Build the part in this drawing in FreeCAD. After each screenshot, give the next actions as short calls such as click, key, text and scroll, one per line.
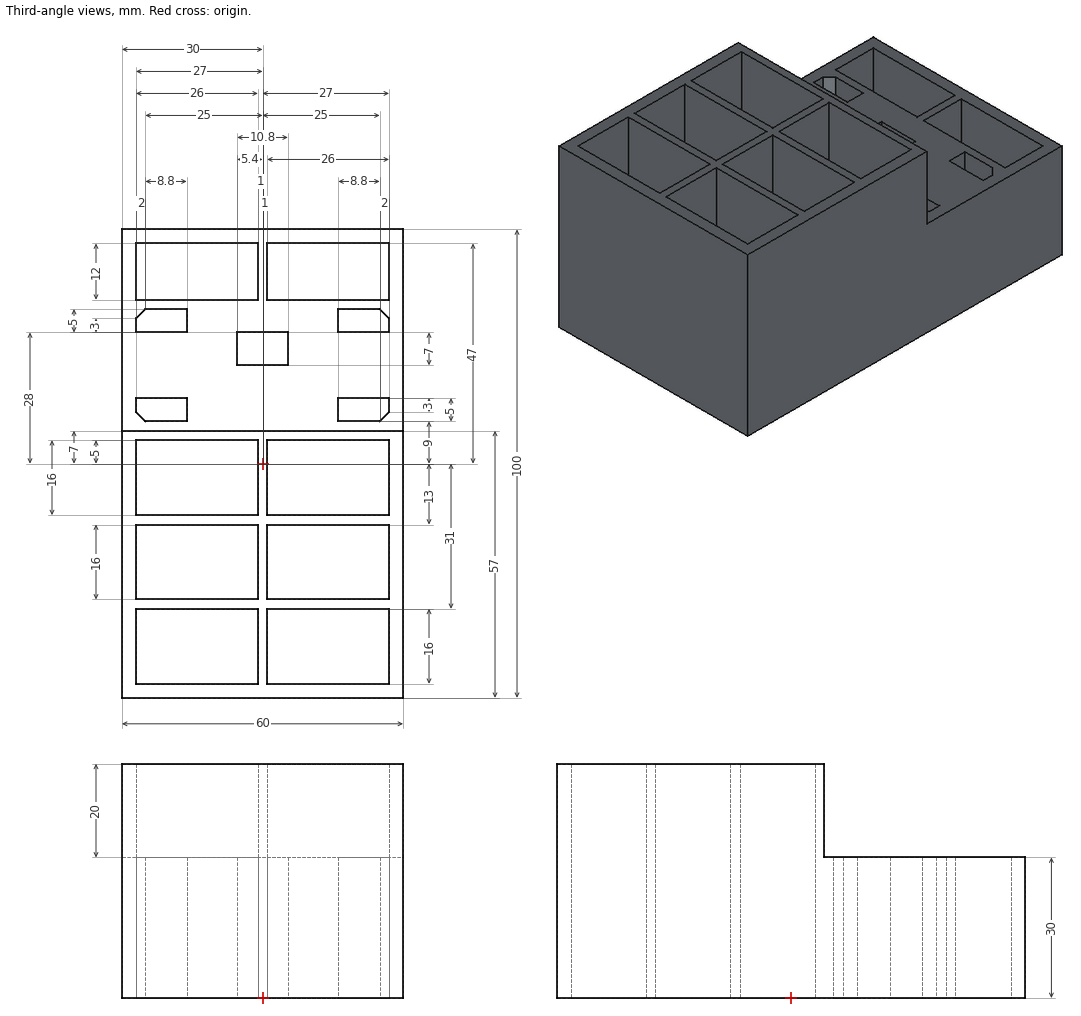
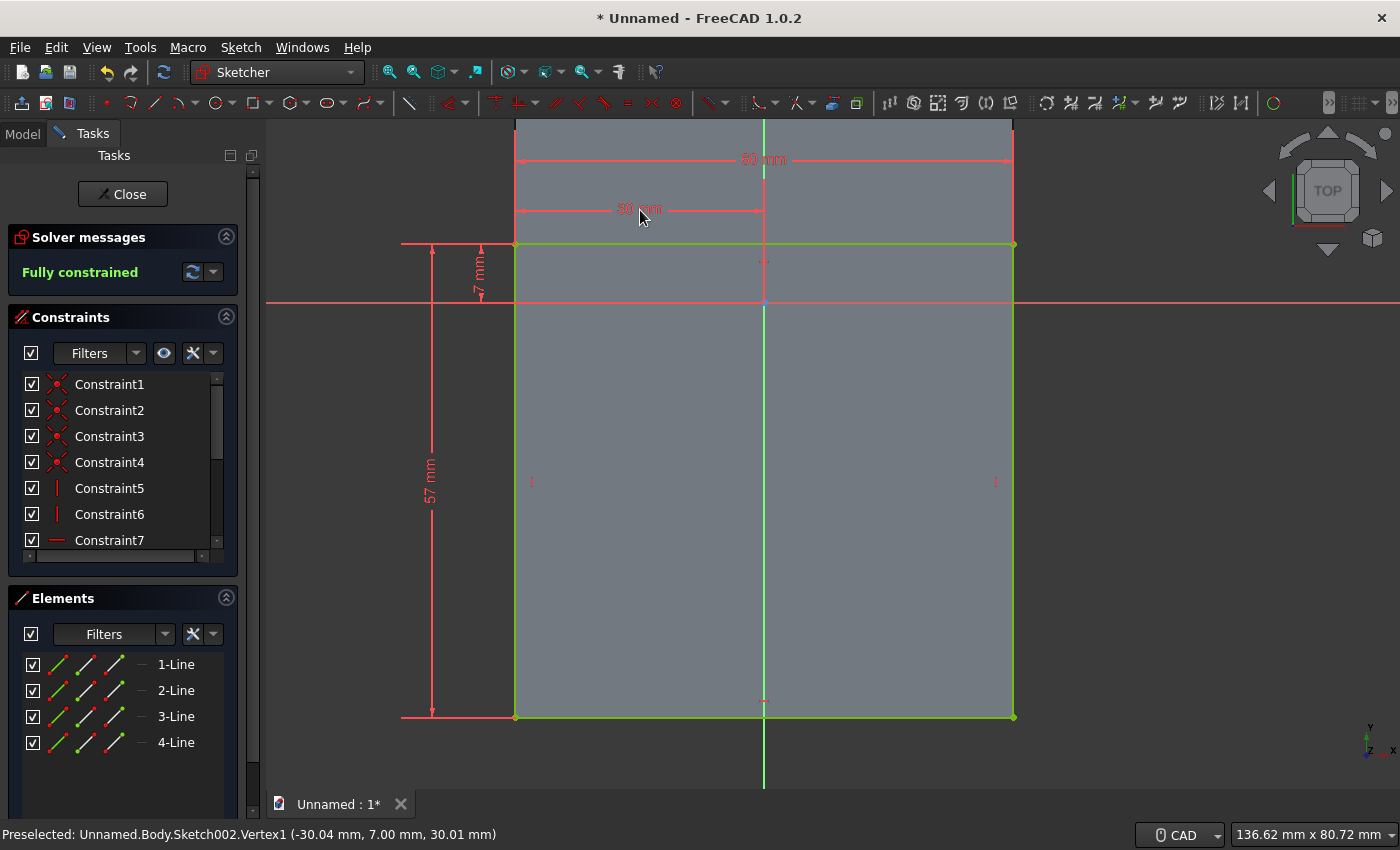
click(123, 194)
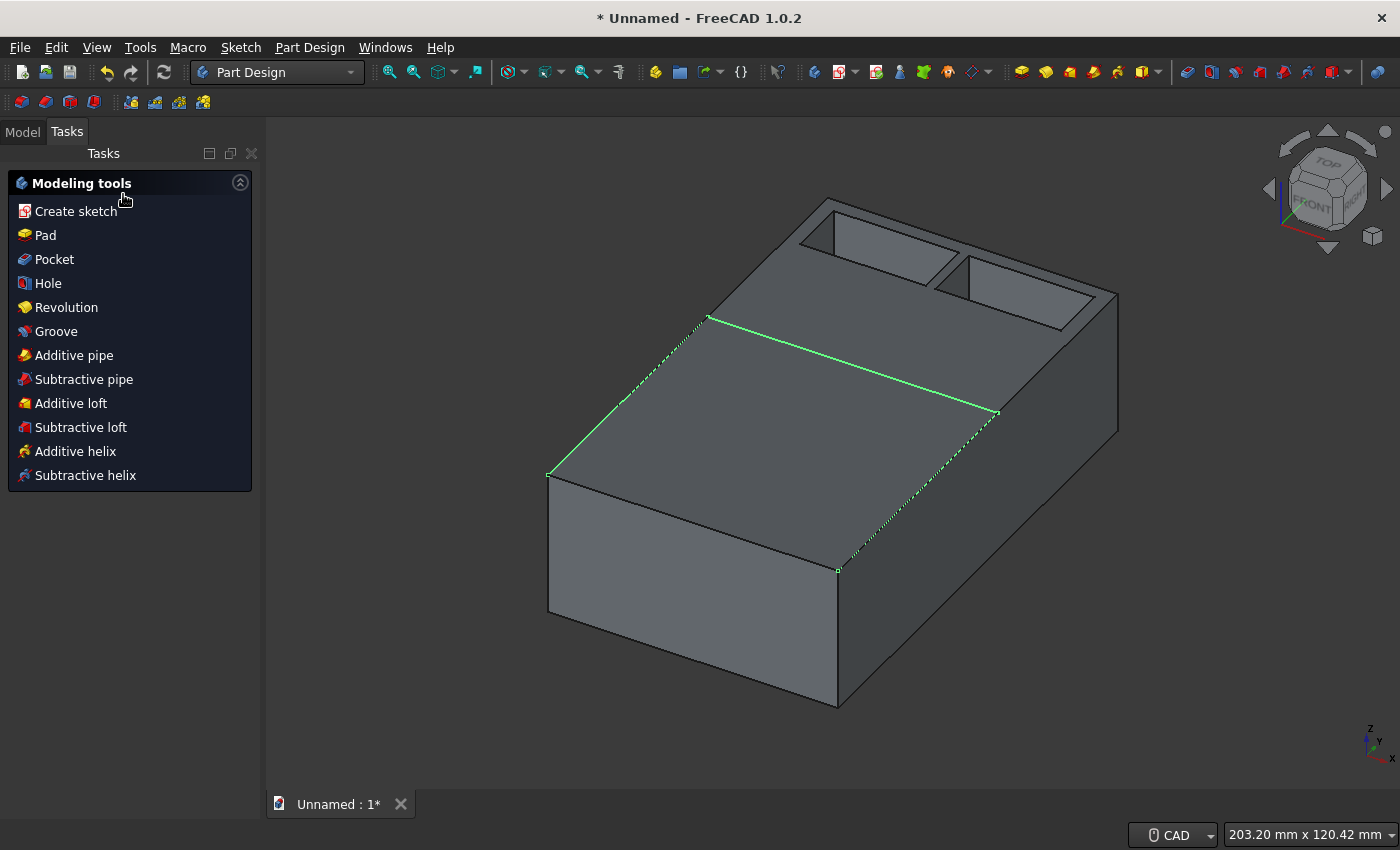
click(1022, 72)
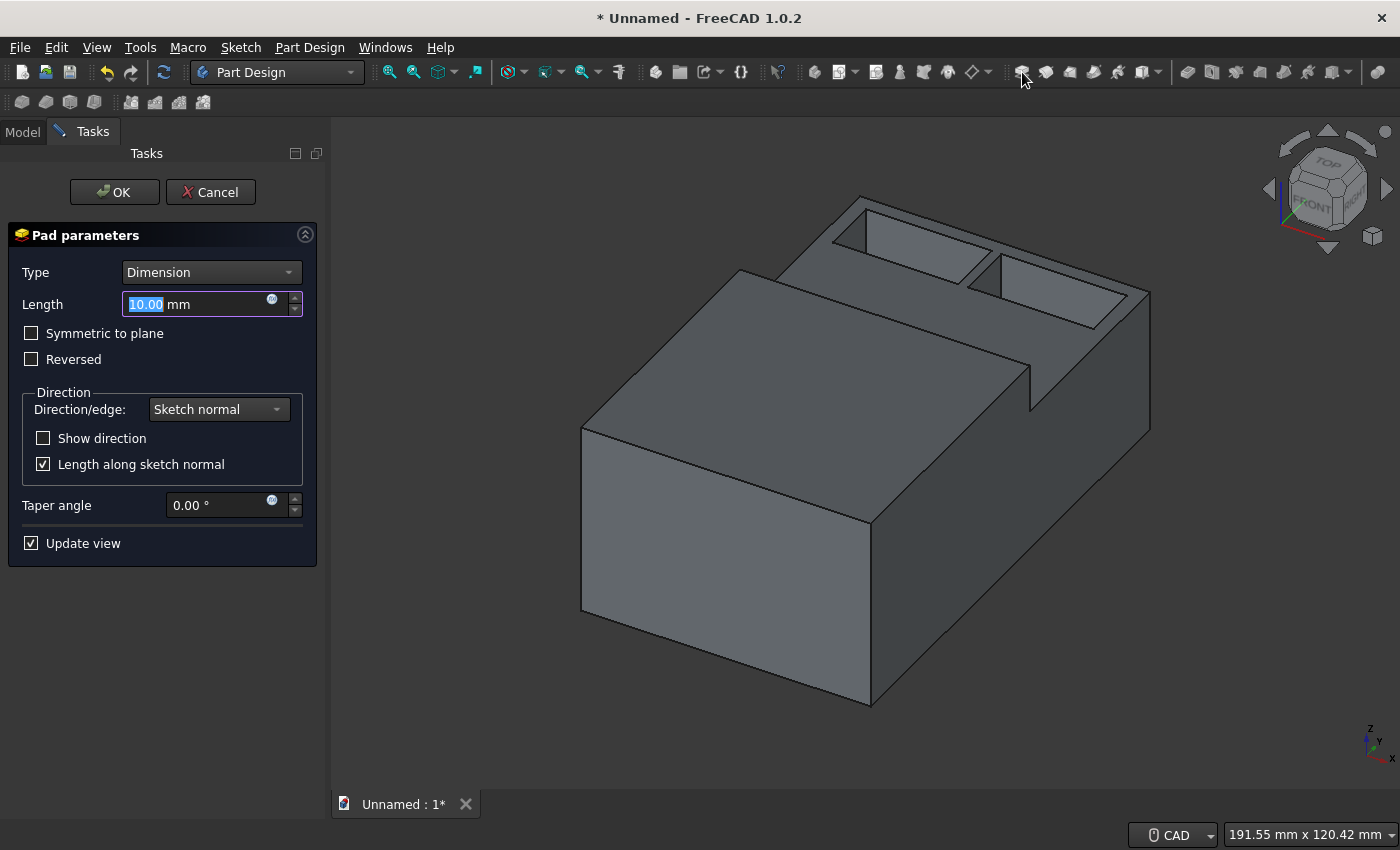
text(20)
key(Tab)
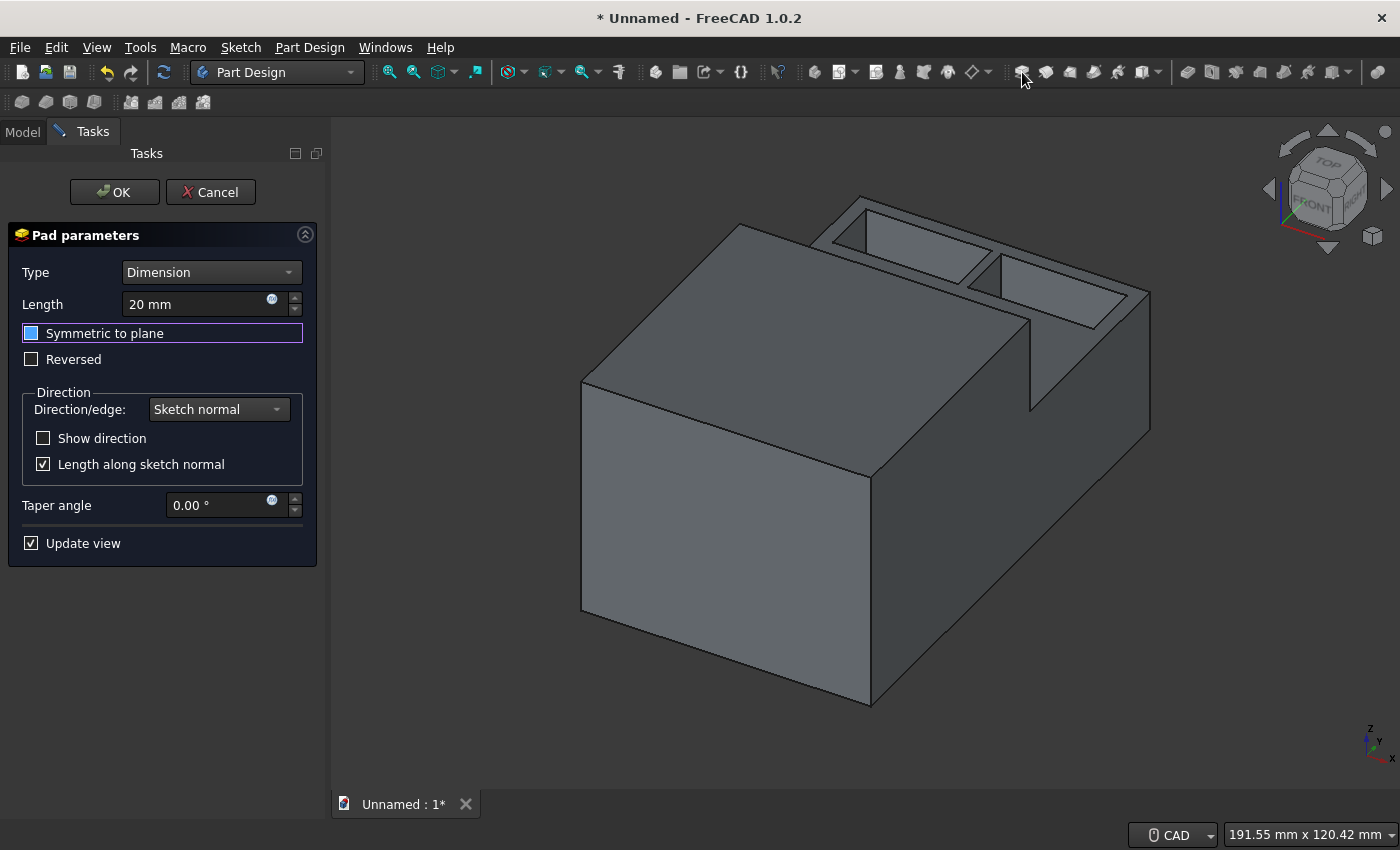
click(115, 192)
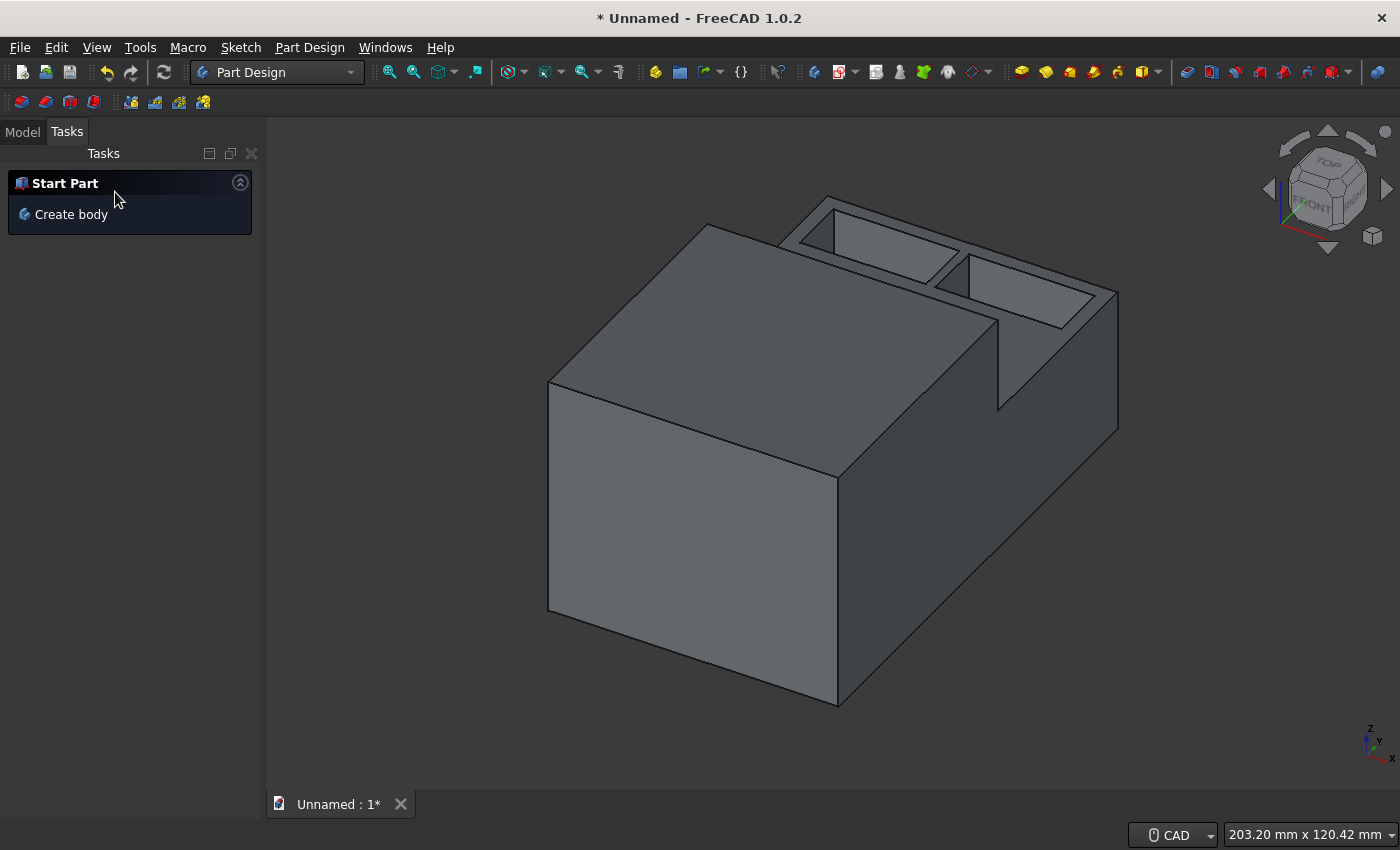
key(v)
key(f)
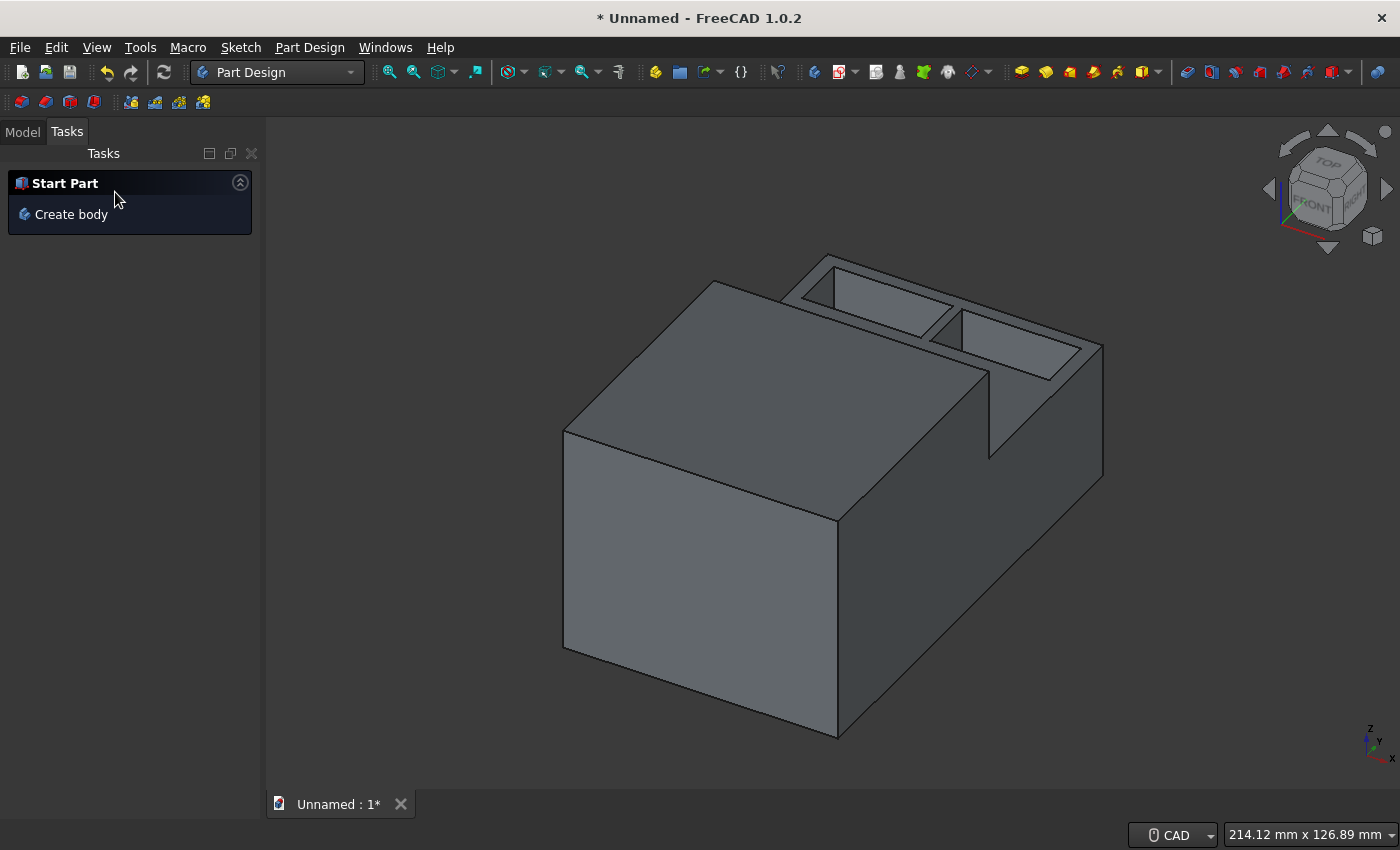
click(776, 400)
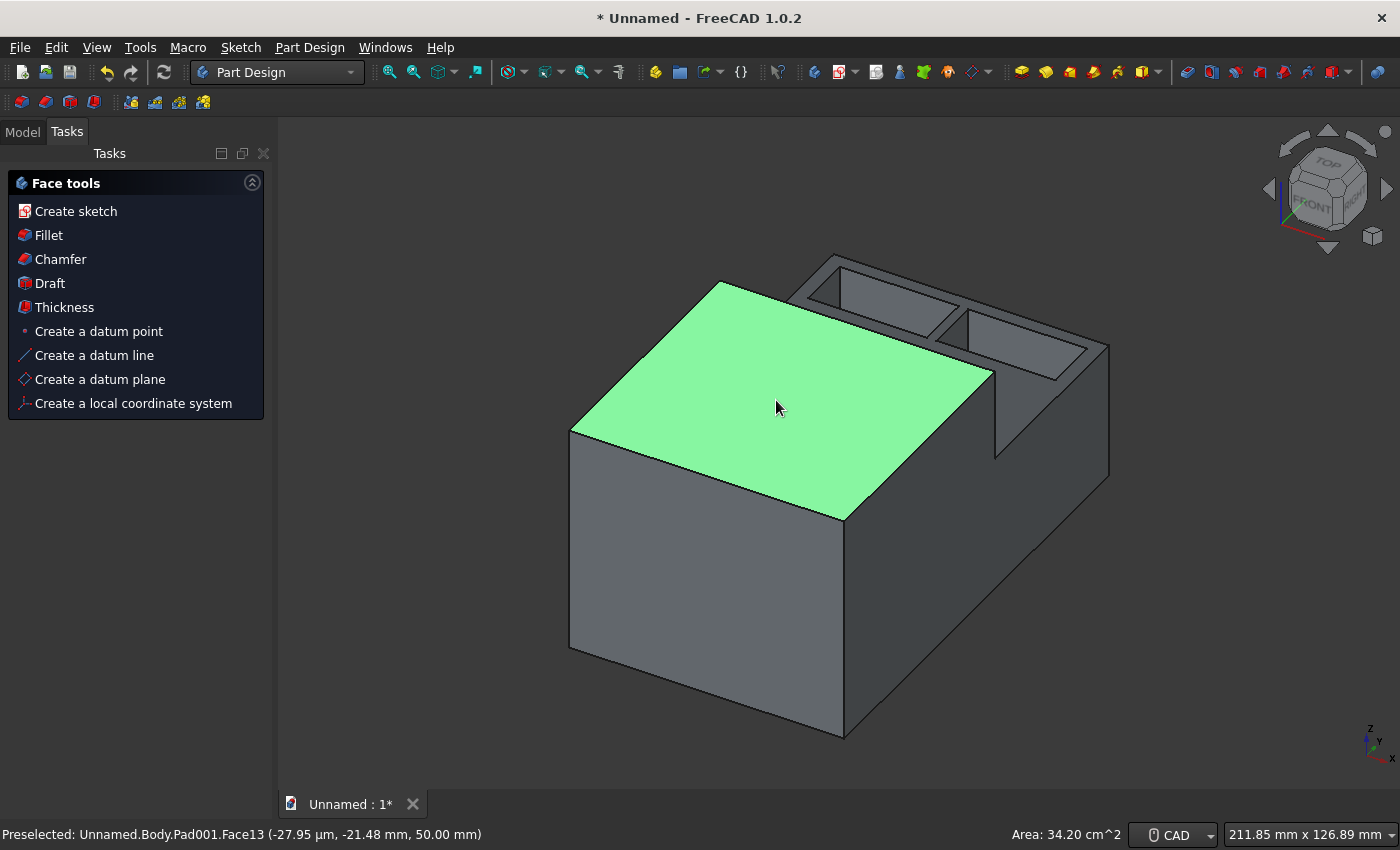
click(840, 72)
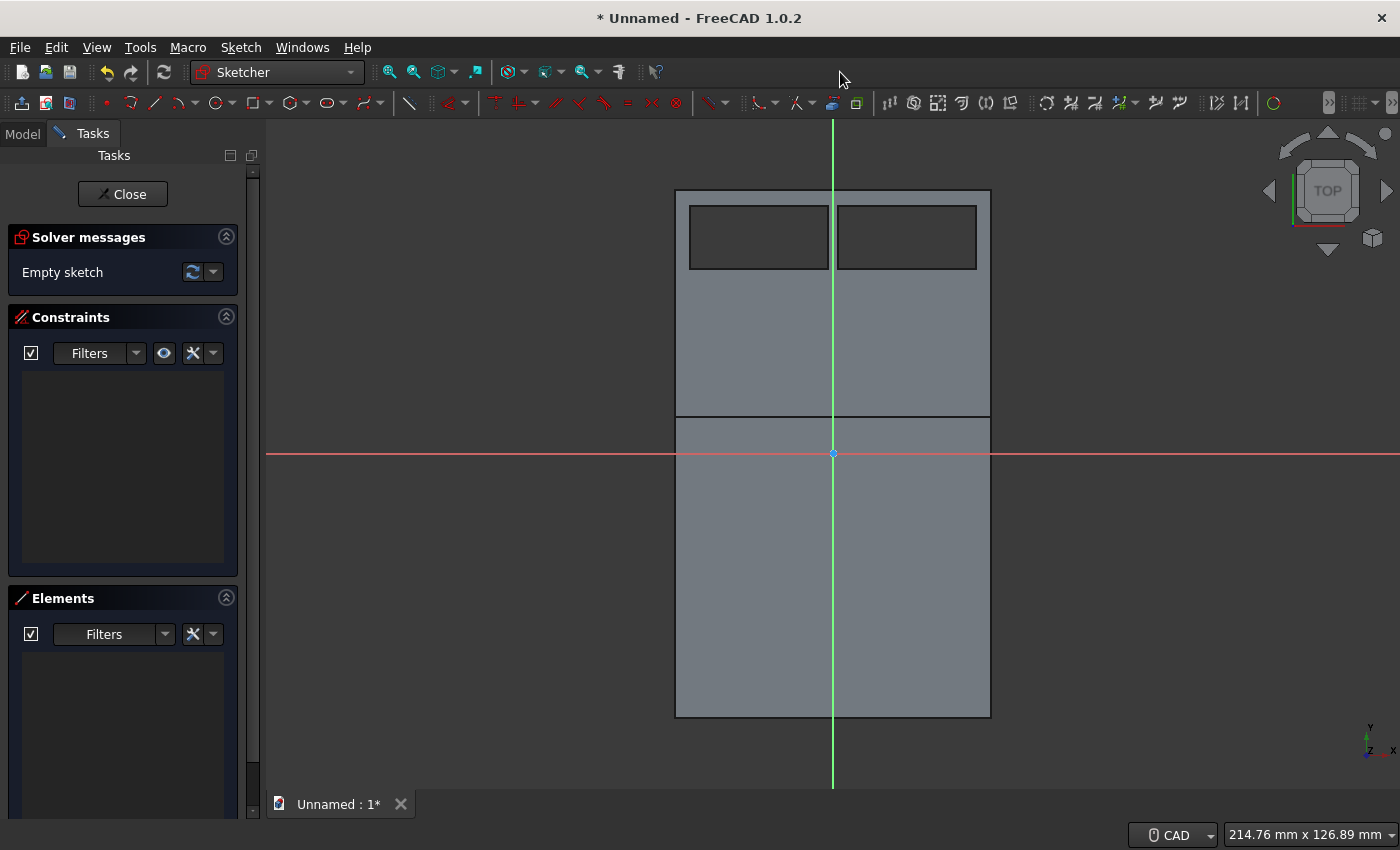
scroll(972, 761, up, 2)